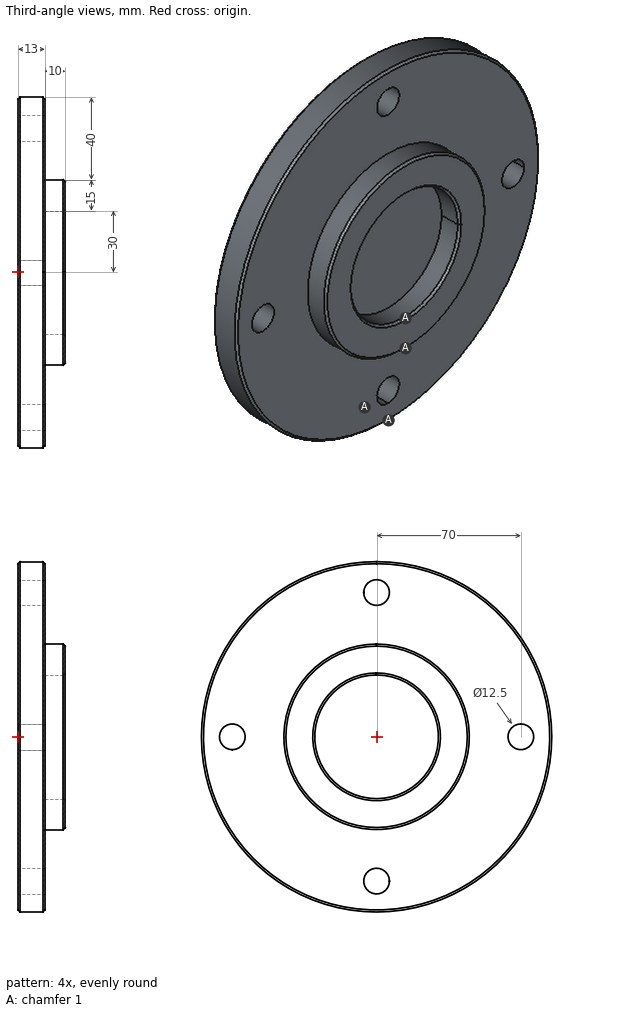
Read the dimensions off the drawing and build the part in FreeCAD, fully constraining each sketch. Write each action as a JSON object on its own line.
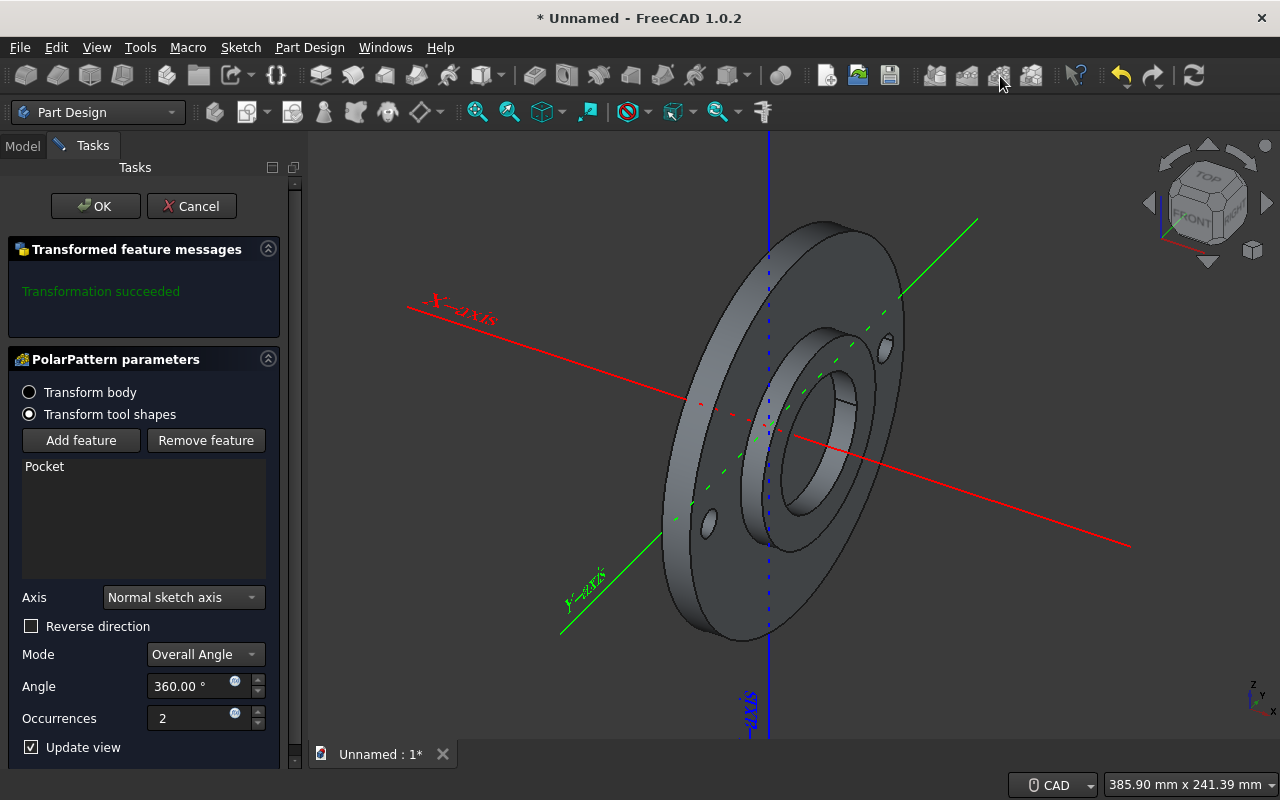
{"action": "left_click", "coordinate": [184, 598]}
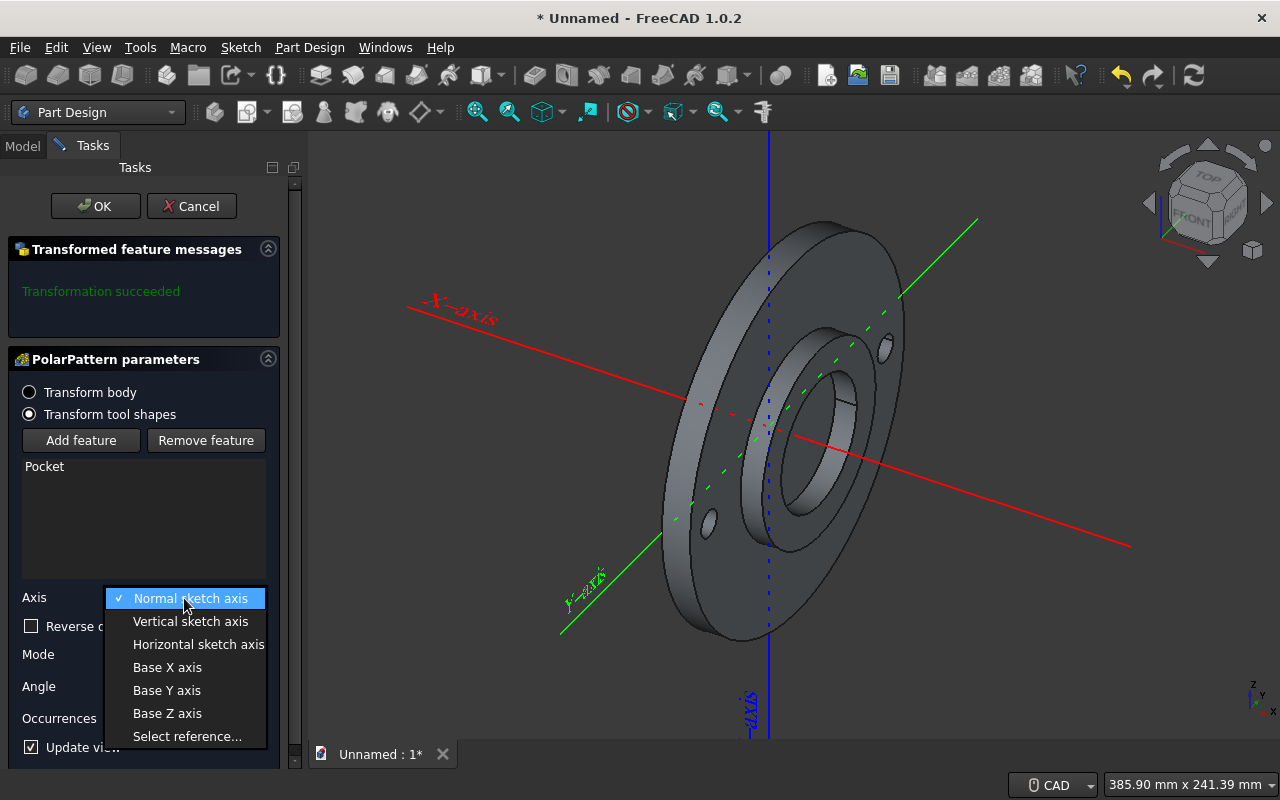
{"action": "left_click", "coordinate": [184, 668]}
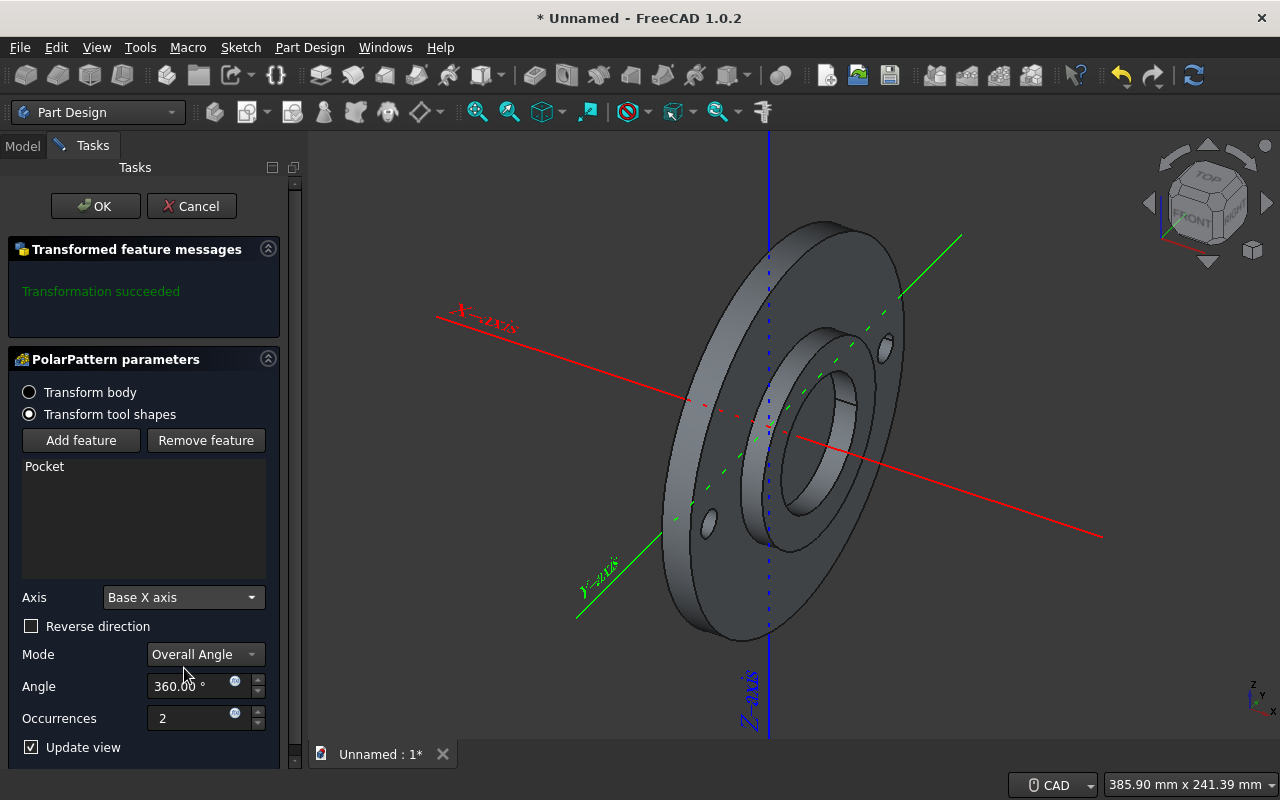
{"action": "triple_click", "coordinate": [198, 718]}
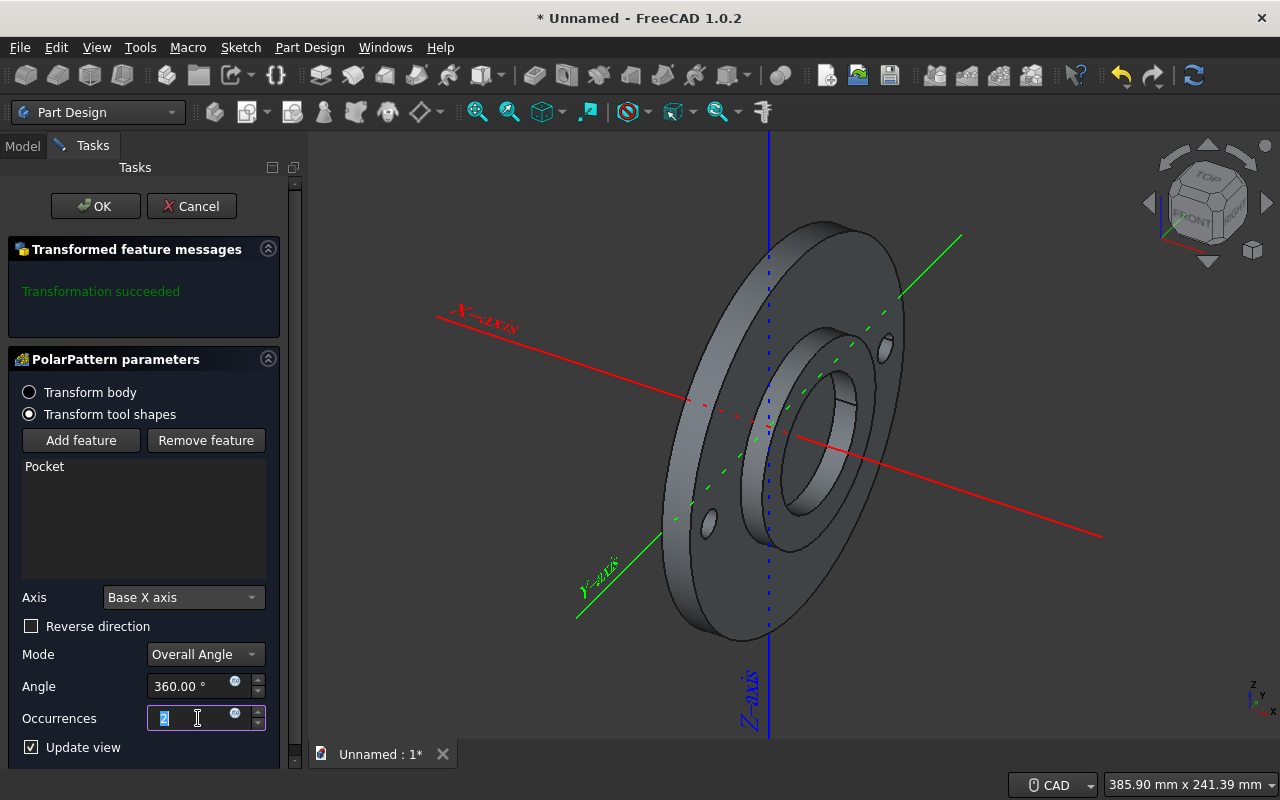
{"action": "type", "text": "4"}
{"action": "key", "text": "Tab"}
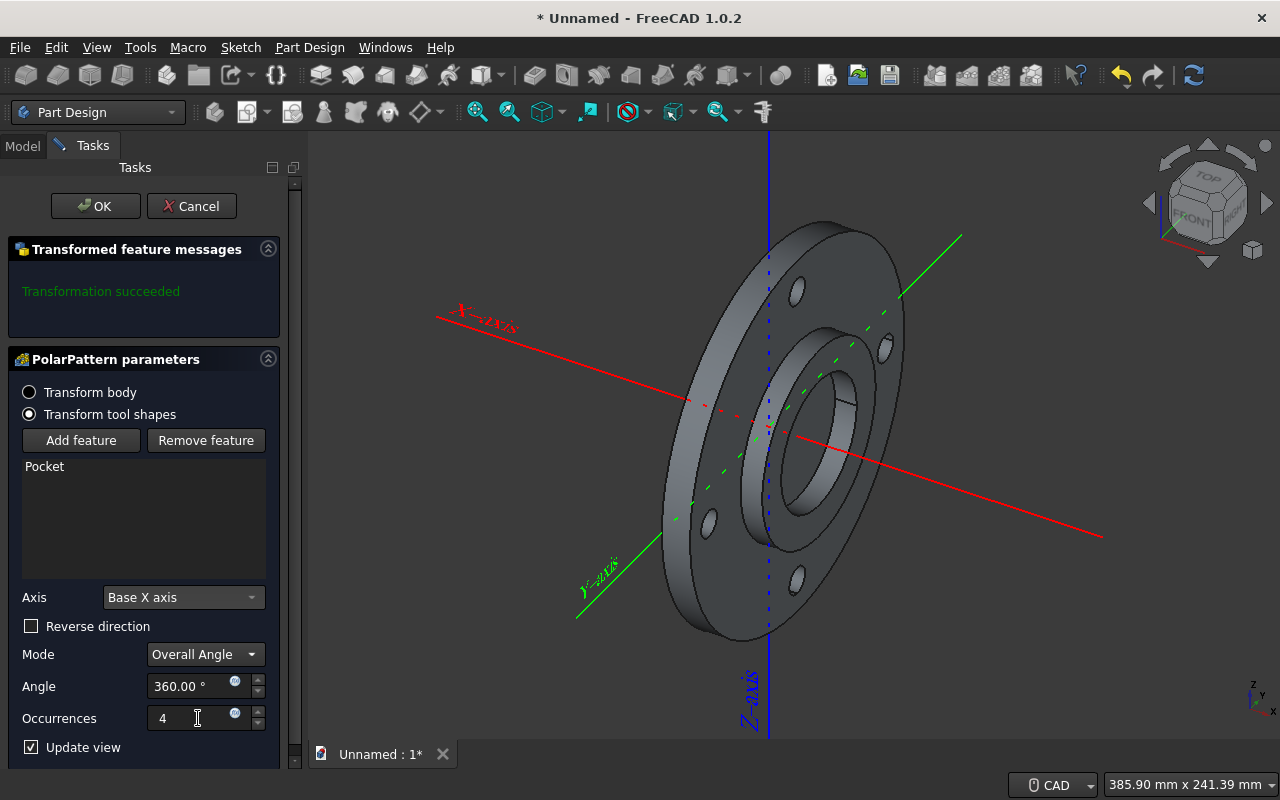
{"action": "left_click", "coordinate": [96, 206]}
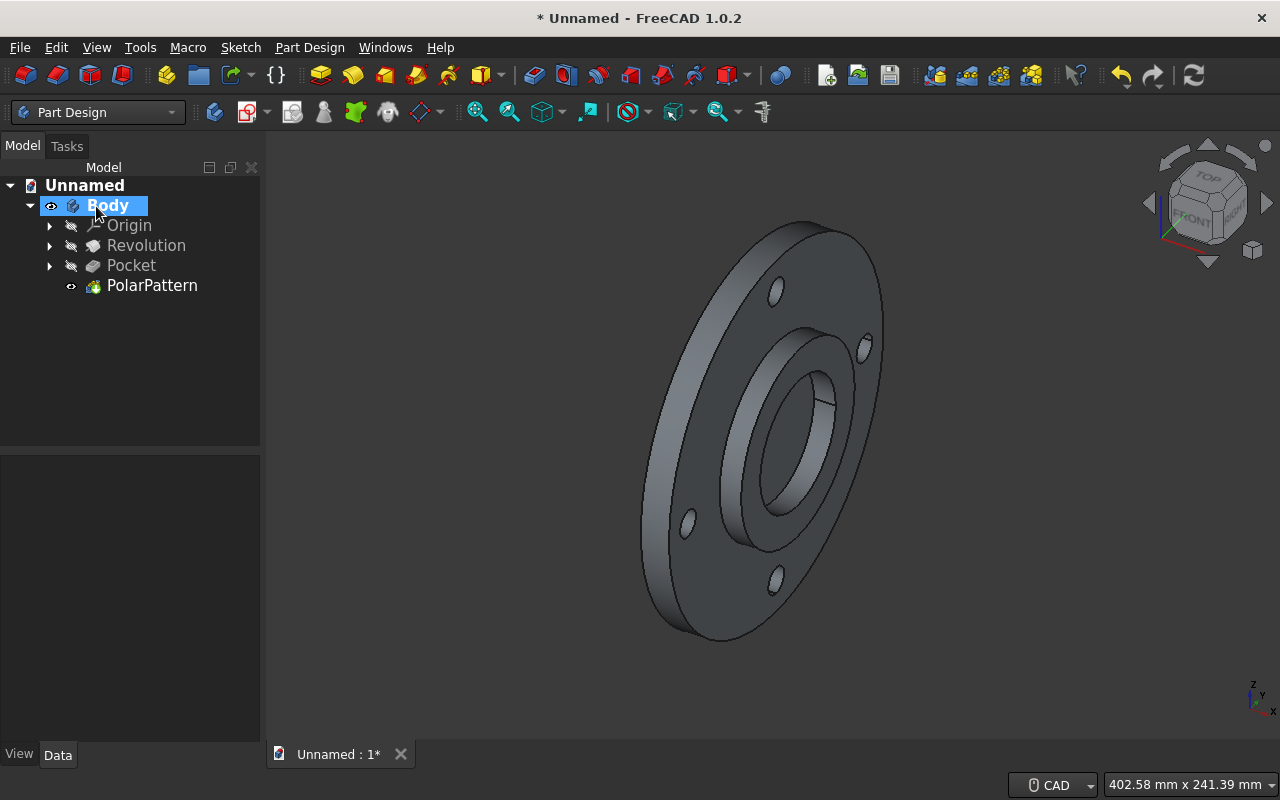
{"action": "left_click", "coordinate": [786, 513]}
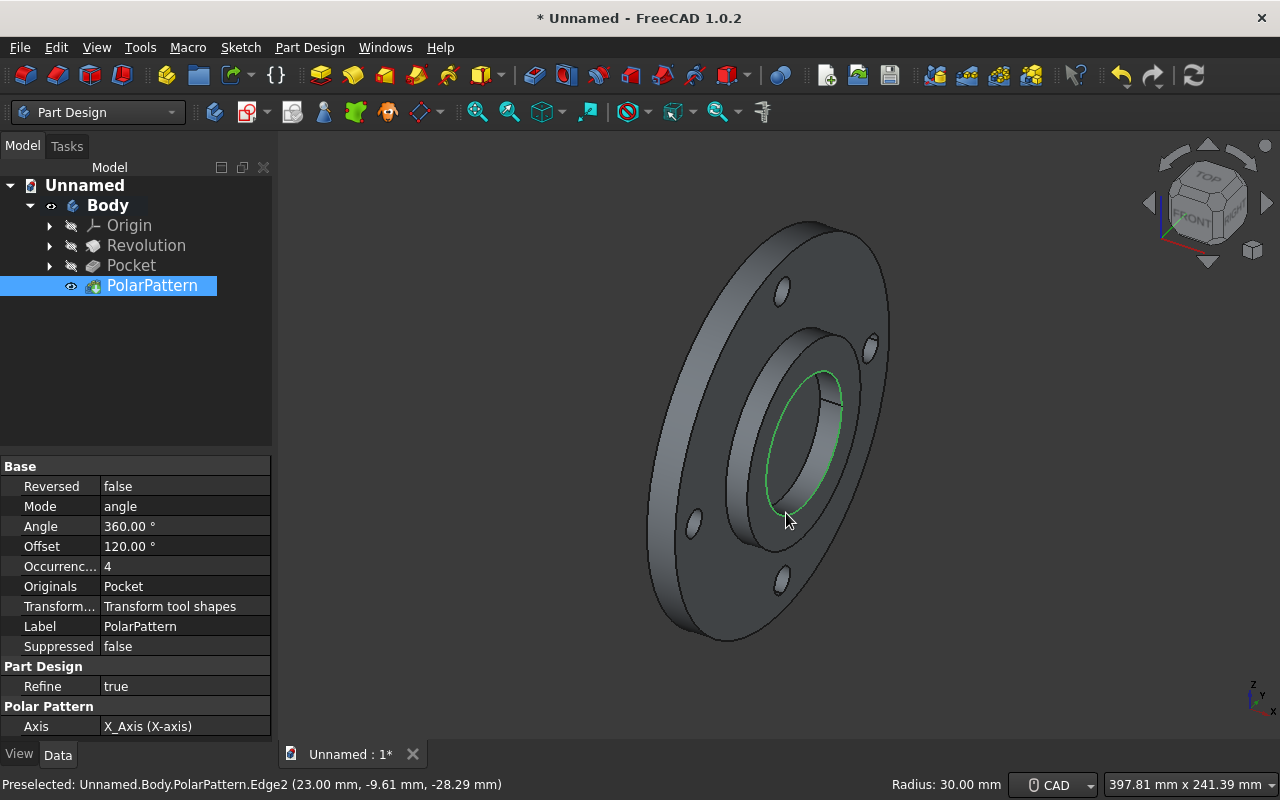
{"action": "left_click", "coordinate": [747, 499], "text": "ctrl"}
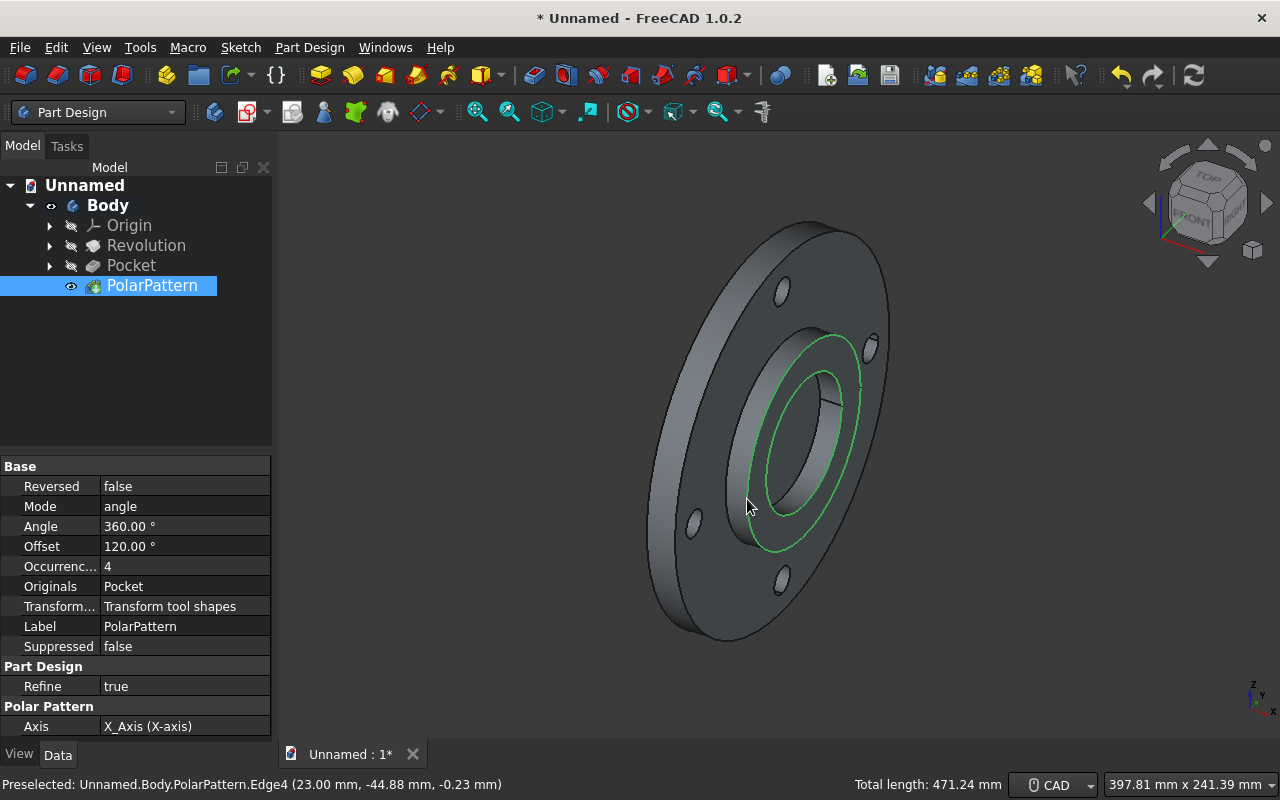
{"action": "left_click", "coordinate": [675, 542], "text": "ctrl"}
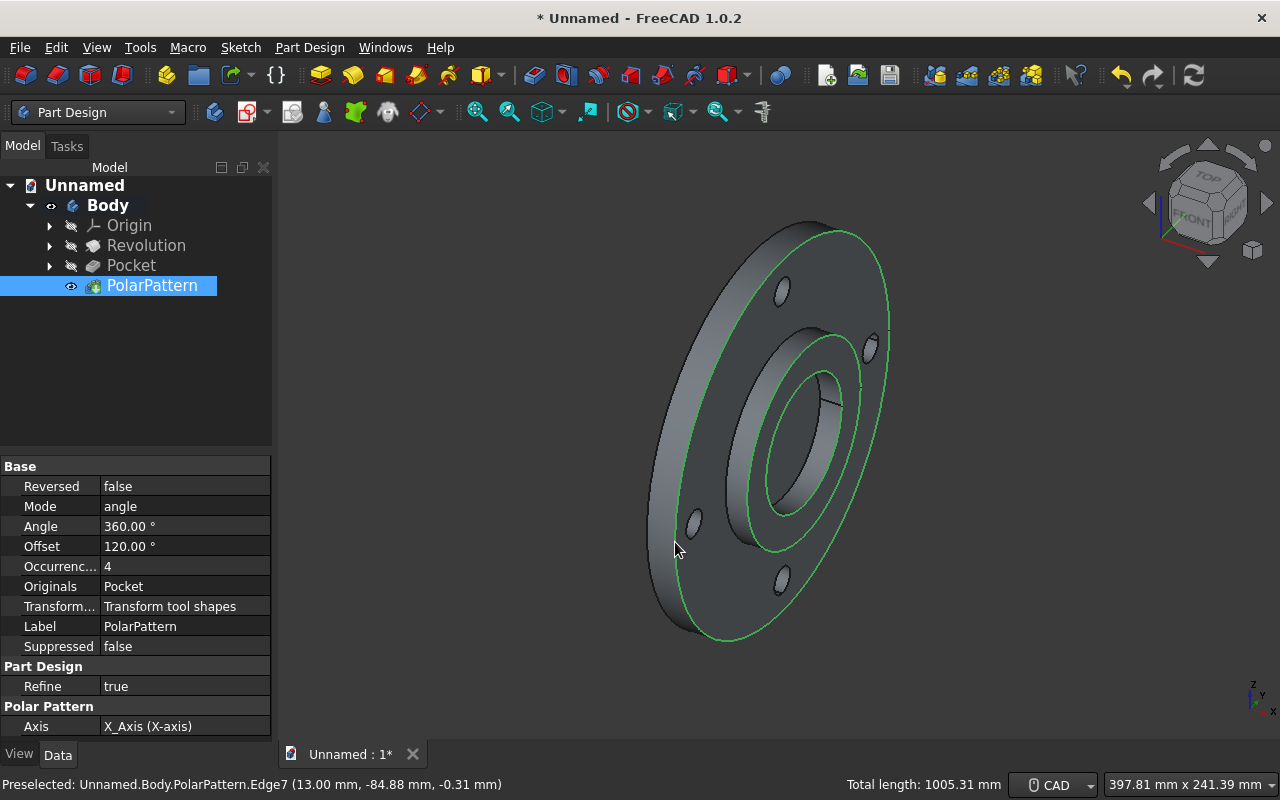
{"action": "key", "text": "0"}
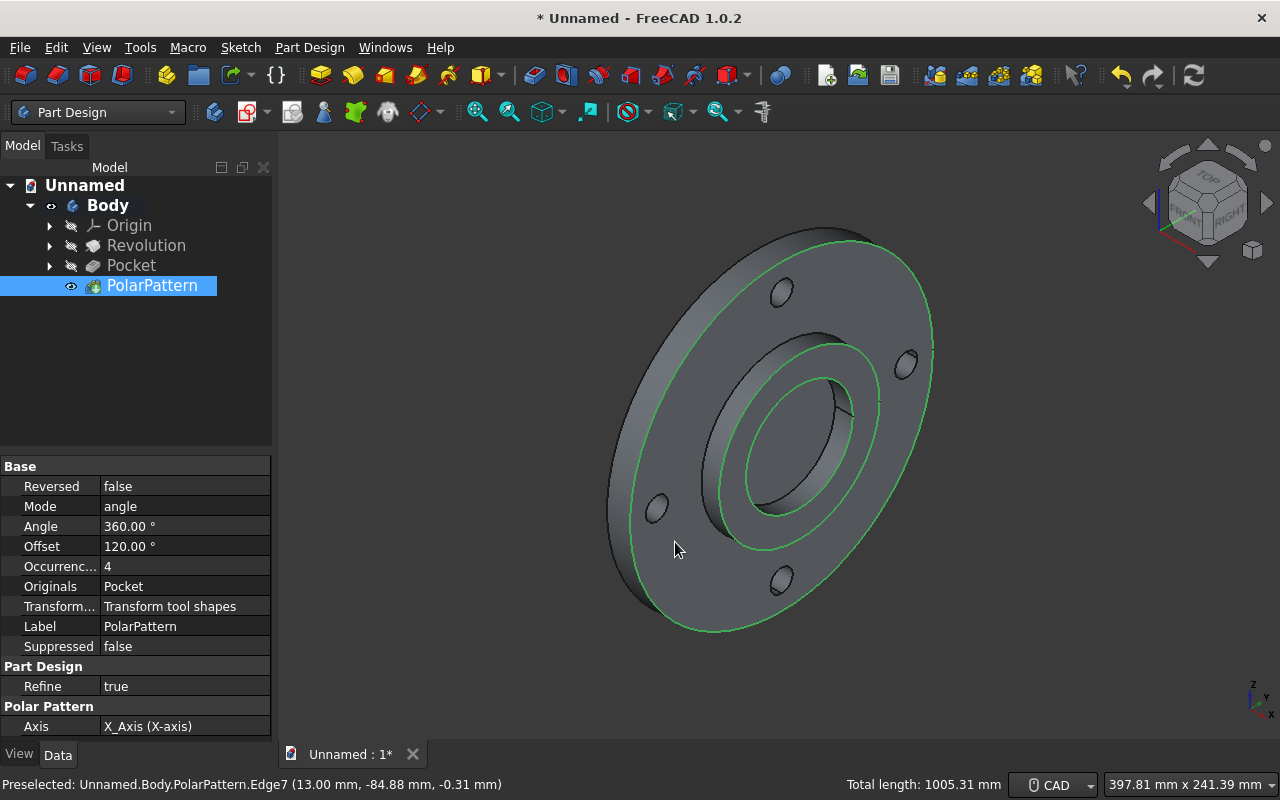
{"action": "key", "text": "2"}